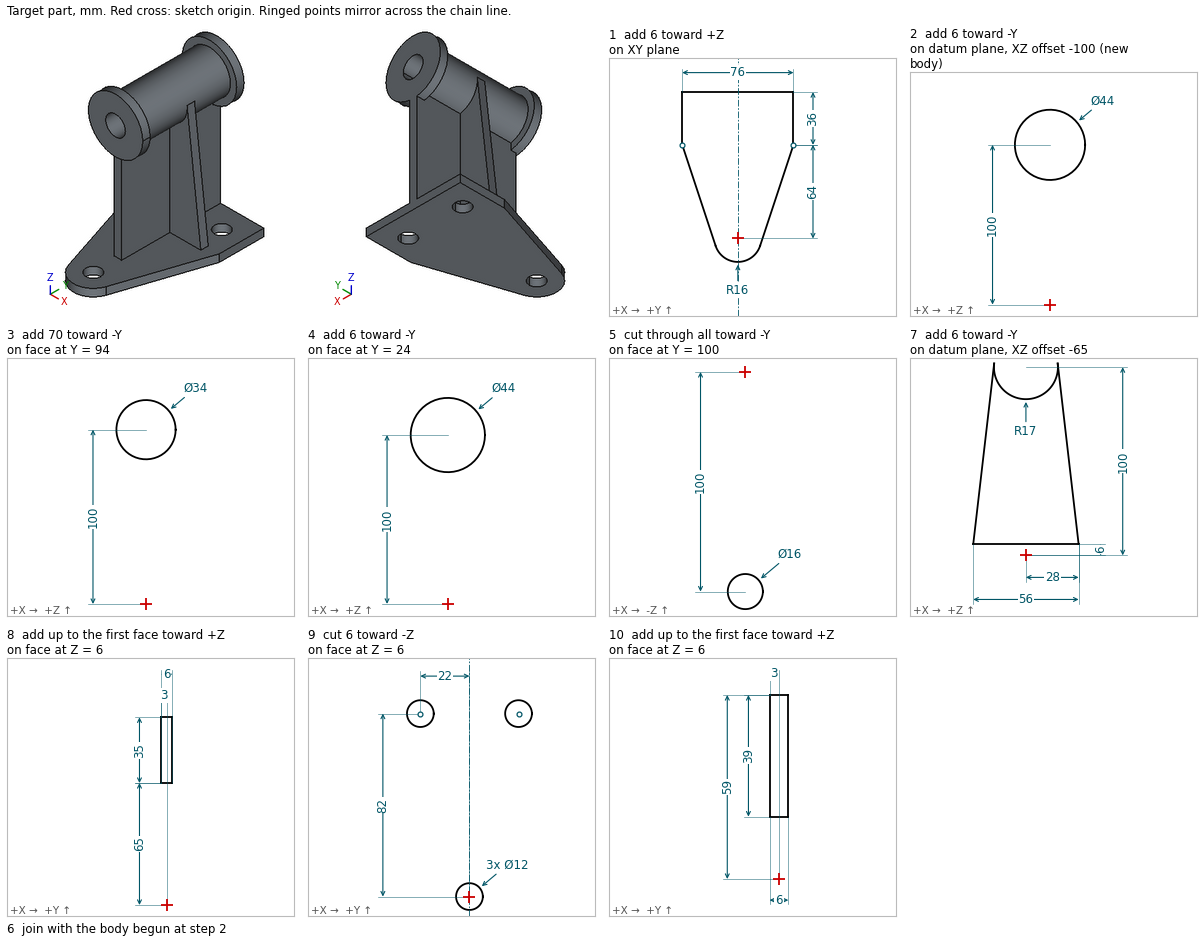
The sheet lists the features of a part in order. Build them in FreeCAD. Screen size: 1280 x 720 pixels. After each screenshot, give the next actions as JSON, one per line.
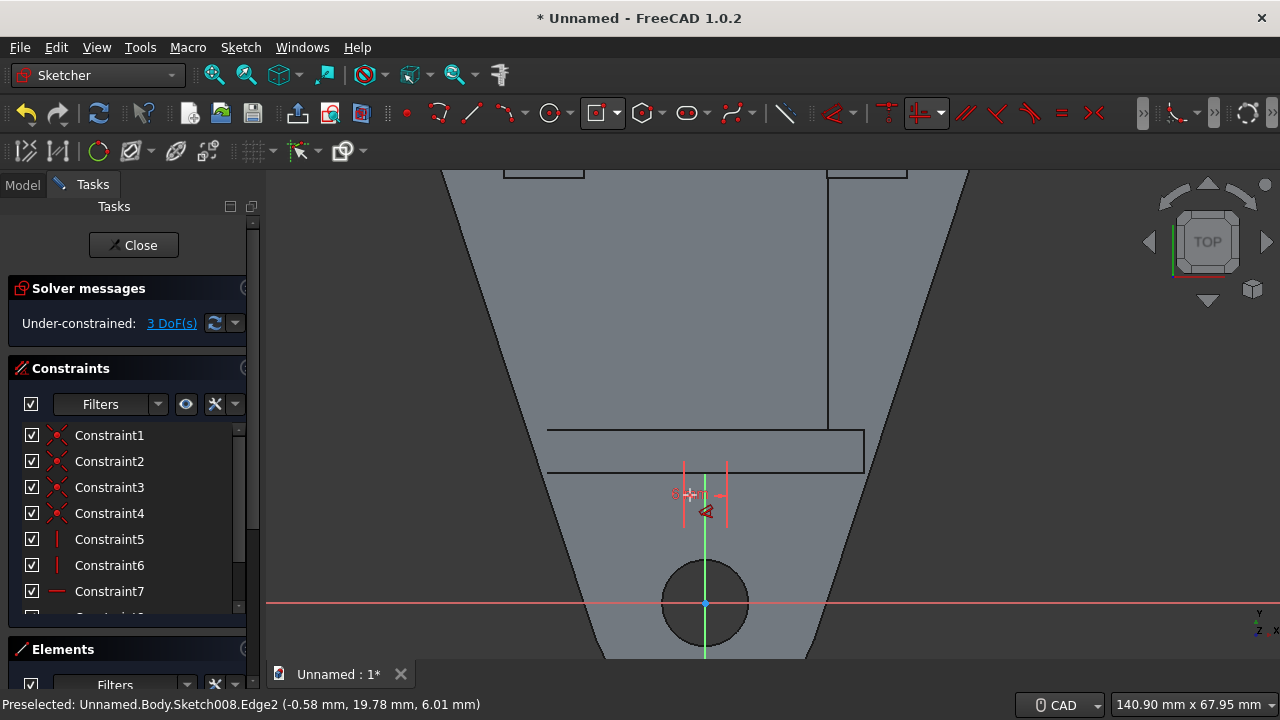
{"action": "left_click", "coordinate": [684, 264]}
{"action": "left_click", "coordinate": [650, 329]}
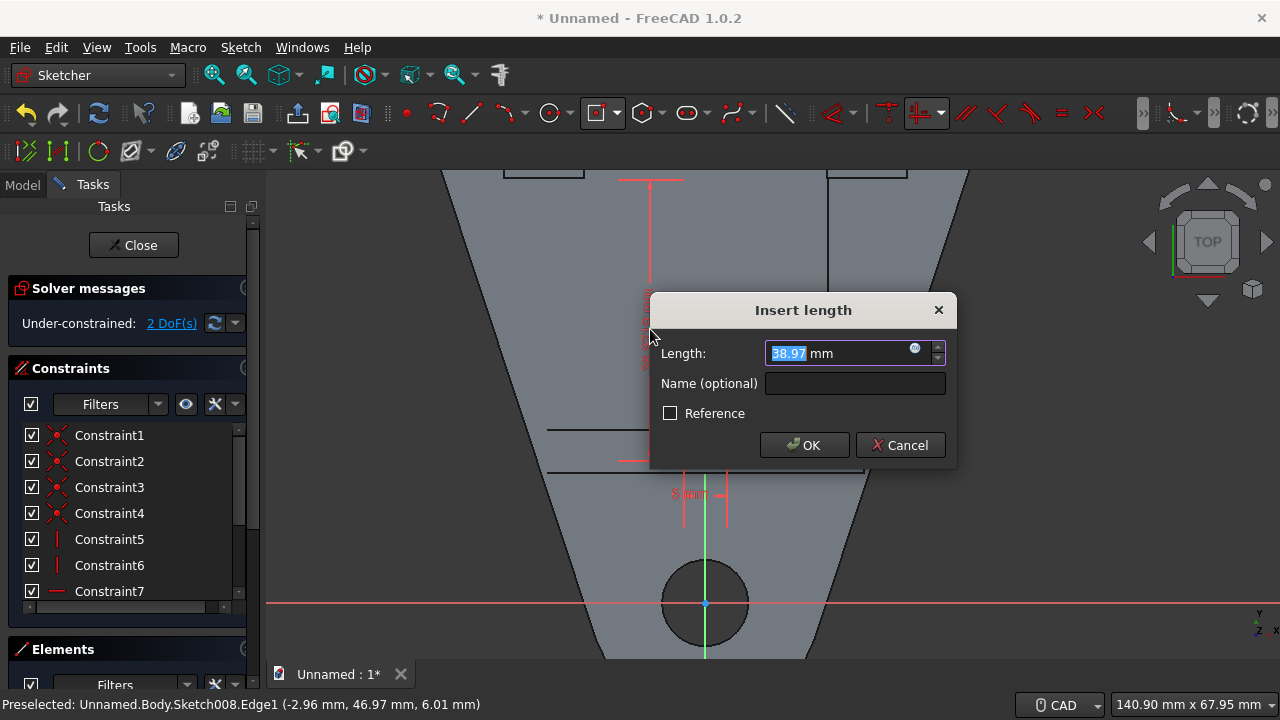
{"action": "type", "text": "39"}
{"action": "key", "text": "Return"}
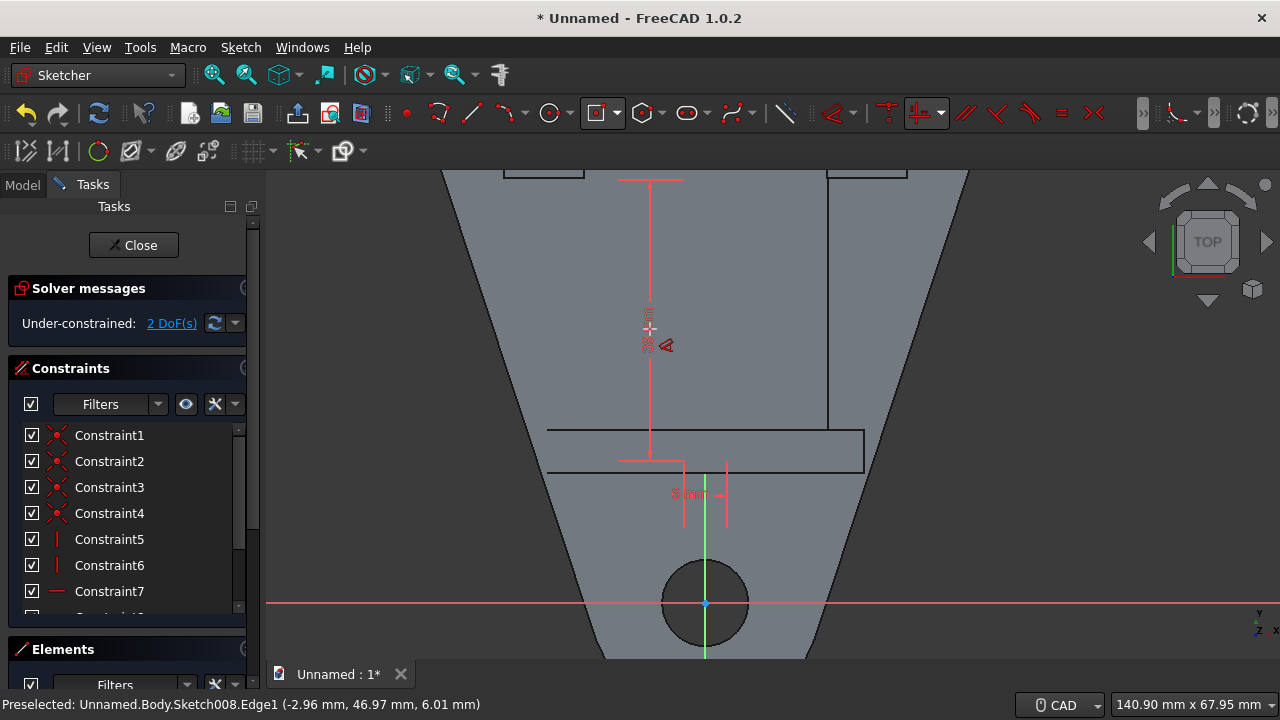
{"action": "scroll", "coordinate": [703, 463], "scroll_direction": "down", "scroll_amount": 2}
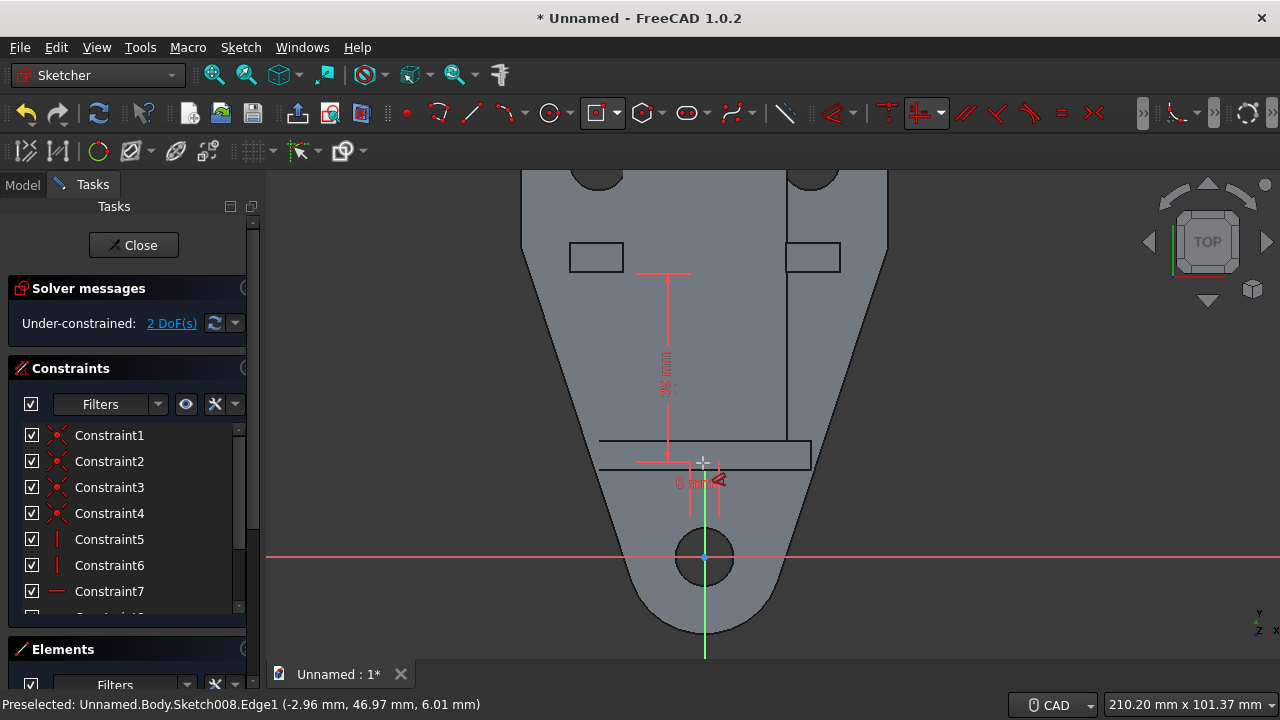
{"action": "scroll", "coordinate": [690, 274], "scroll_direction": "up", "scroll_amount": 6}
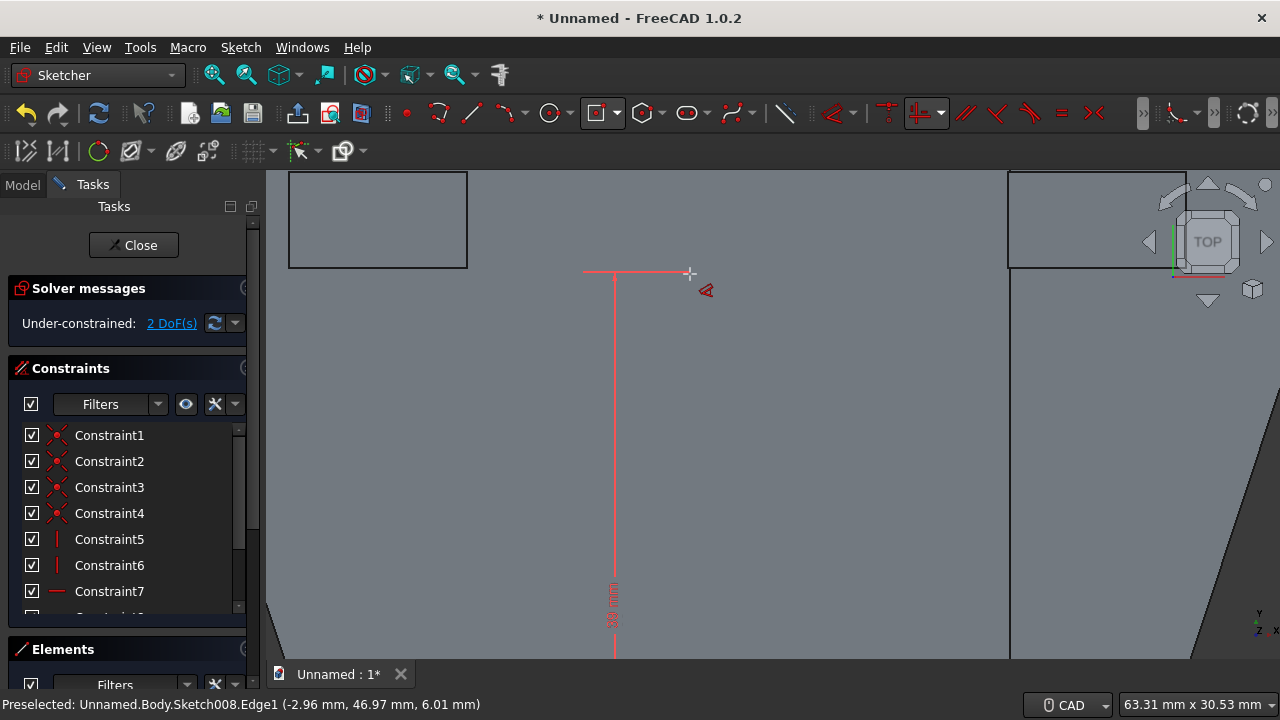
{"action": "left_click", "coordinate": [690, 272]}
{"action": "left_click", "coordinate": [714, 238]}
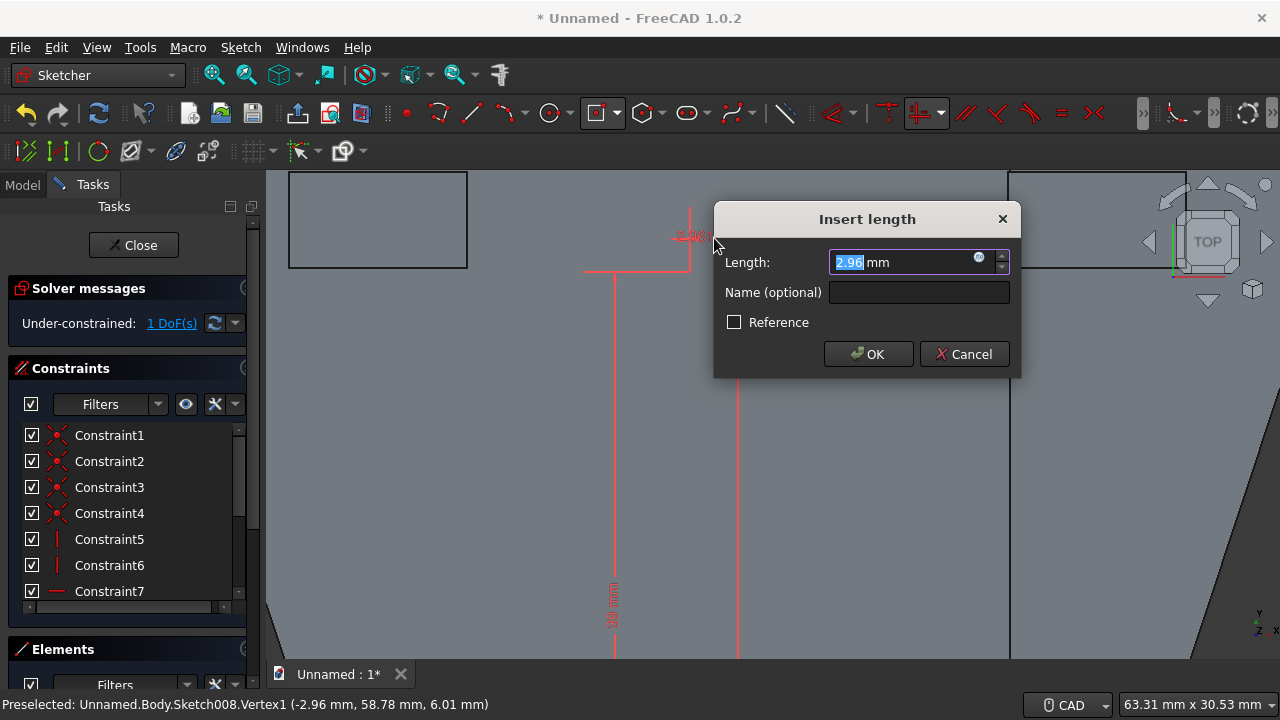
{"action": "type", "text": "3"}
{"action": "key", "text": "Return"}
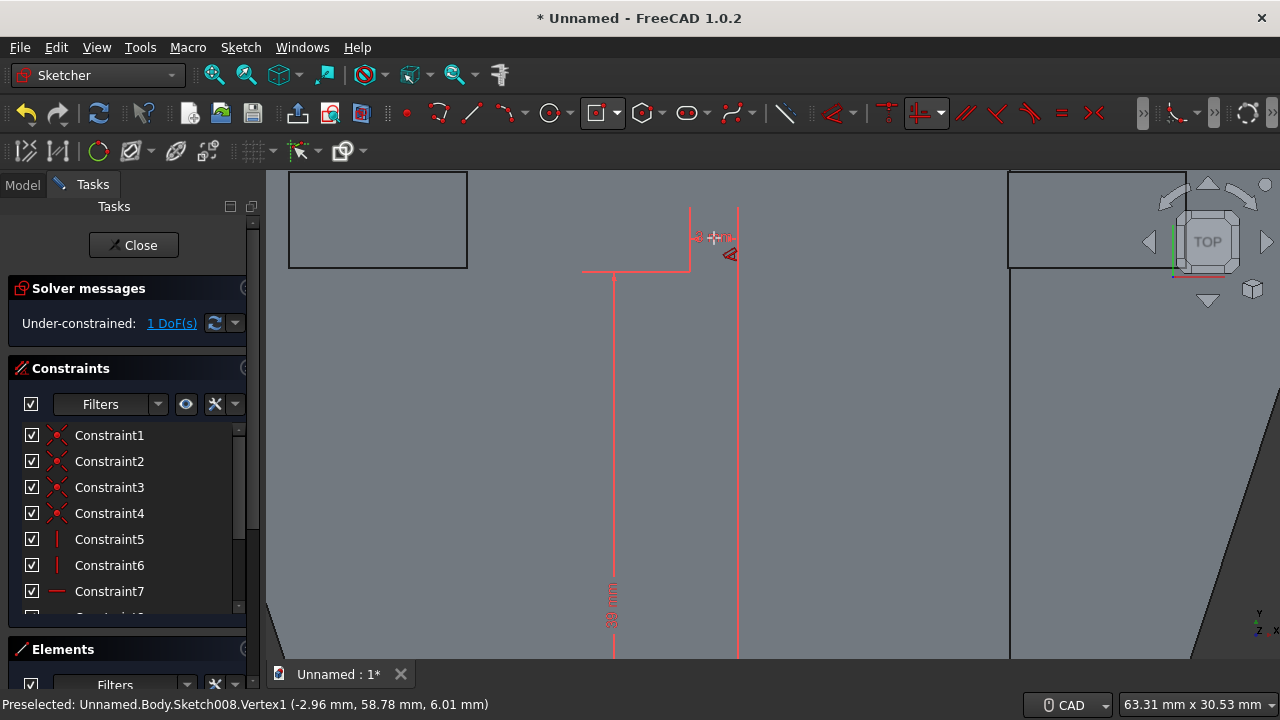
{"action": "left_click", "coordinate": [690, 272]}
{"action": "left_click", "coordinate": [656, 451]}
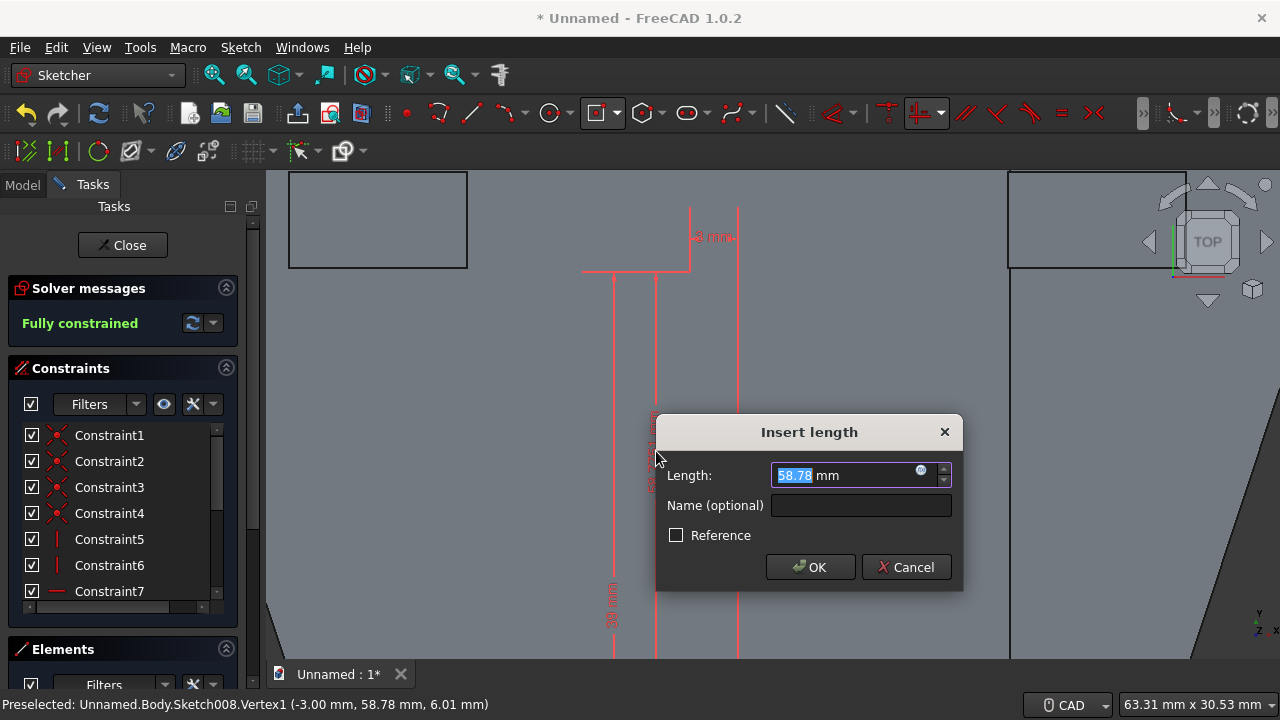
{"action": "type", "text": "59"}
{"action": "key", "text": "Return"}
{"action": "key", "text": "Escape"}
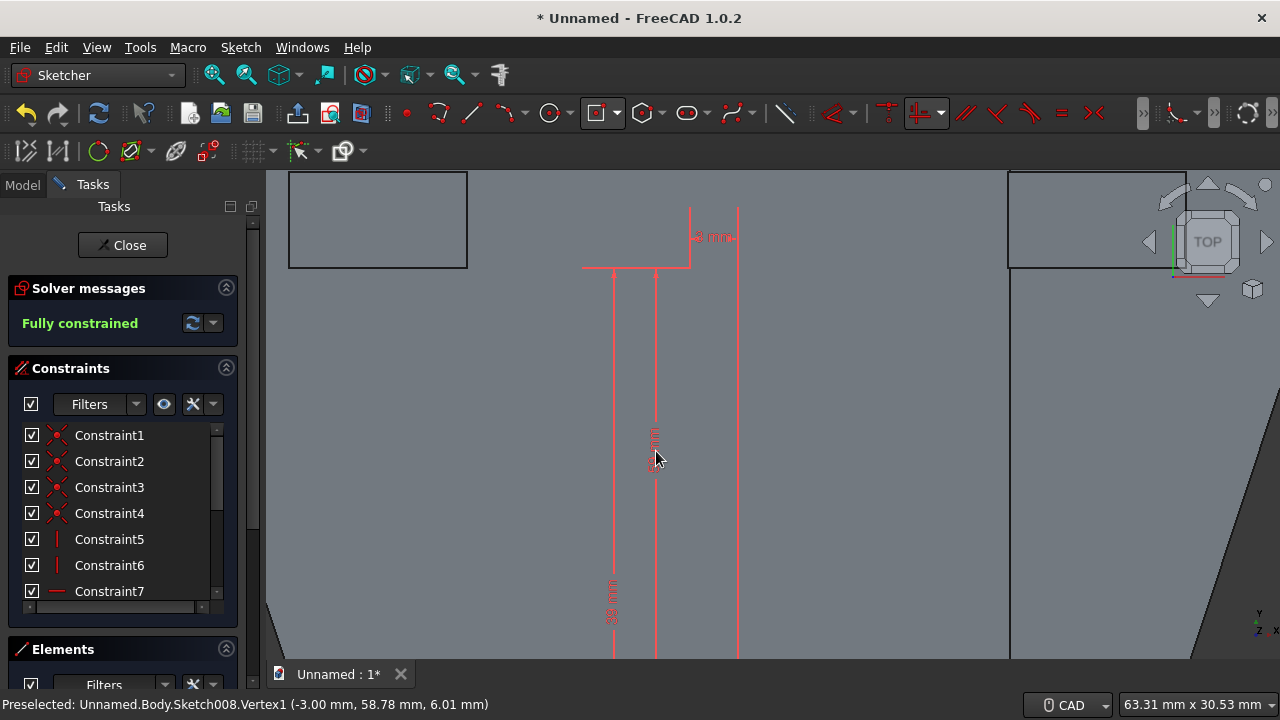
{"action": "left_click", "coordinate": [123, 245]}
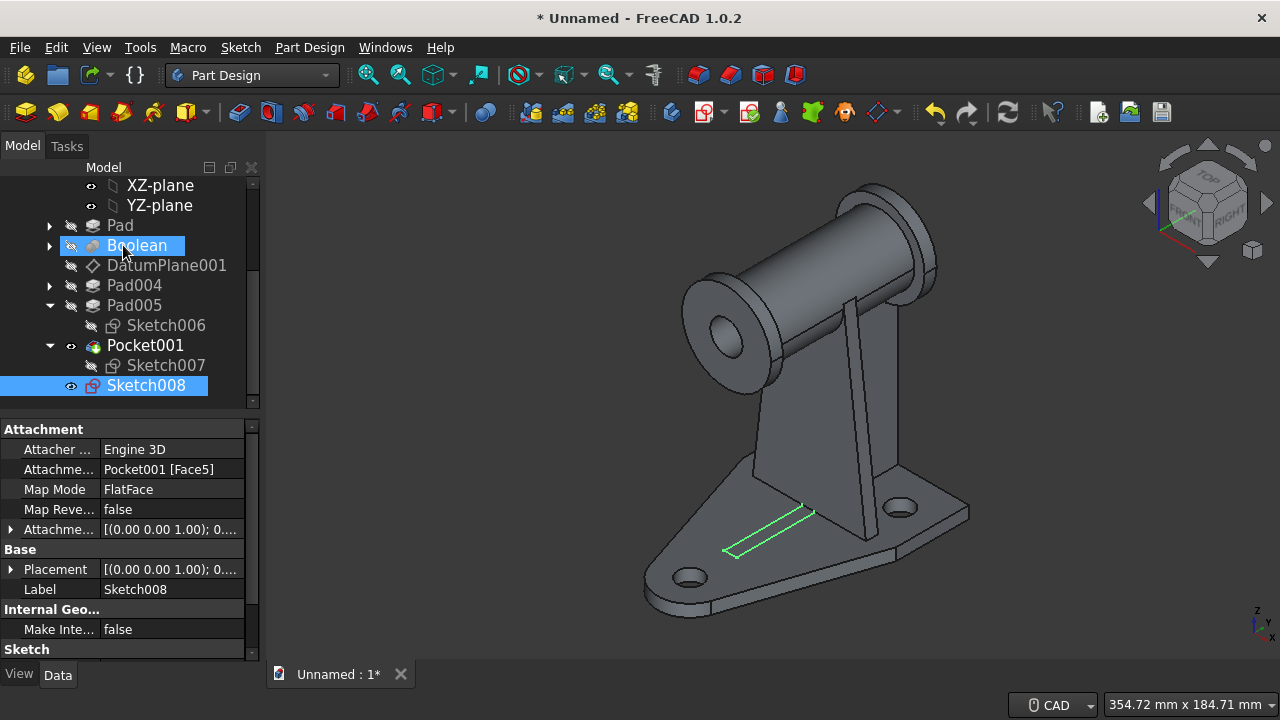
{"action": "left_click", "coordinate": [26, 112]}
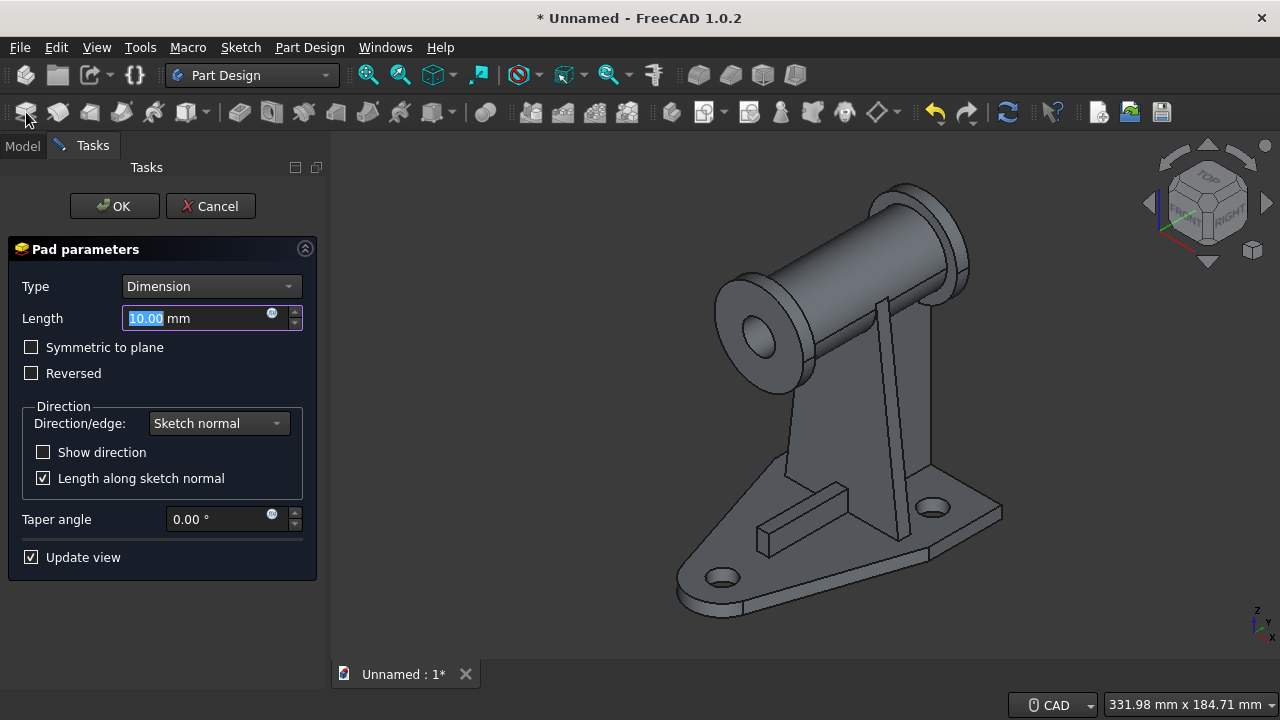
{"action": "left_click", "coordinate": [212, 286]}